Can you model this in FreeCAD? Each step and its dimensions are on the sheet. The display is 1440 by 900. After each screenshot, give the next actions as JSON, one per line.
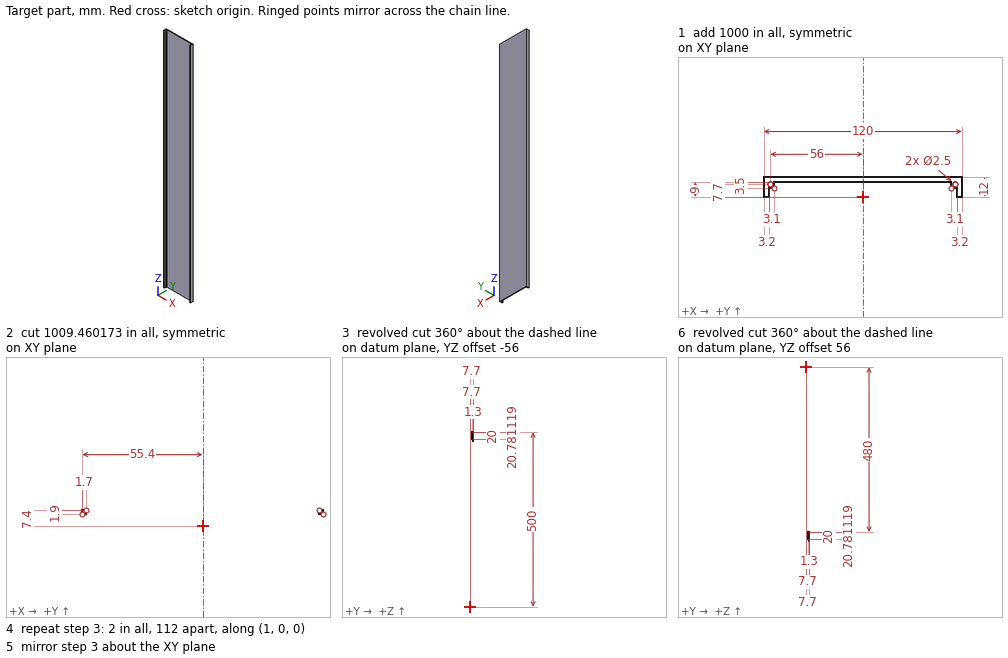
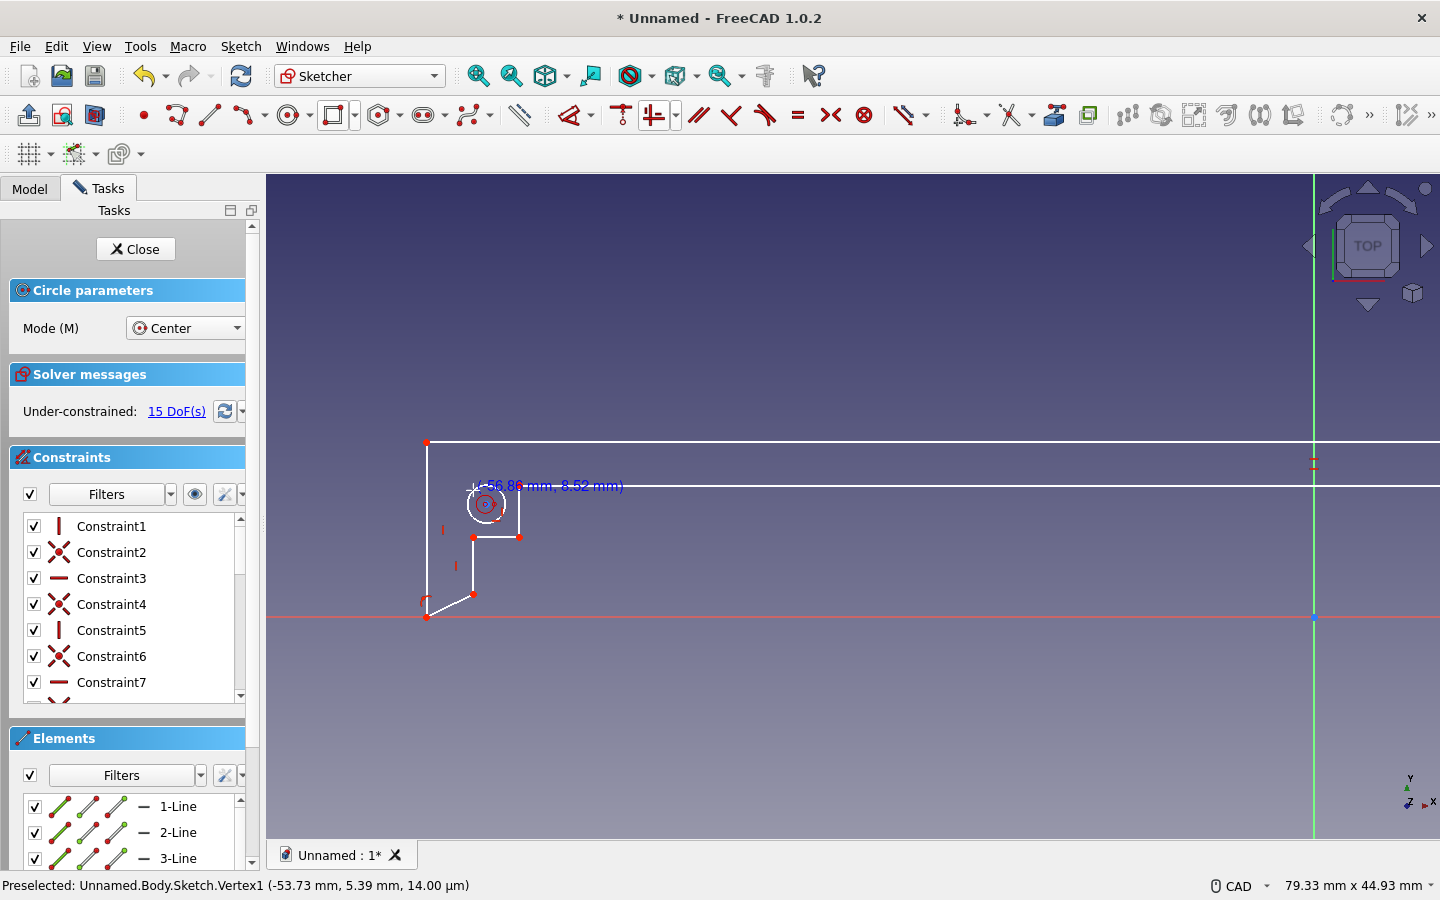
{"action": "scroll", "coordinate": [476, 494], "scroll_direction": "down", "scroll_amount": 5}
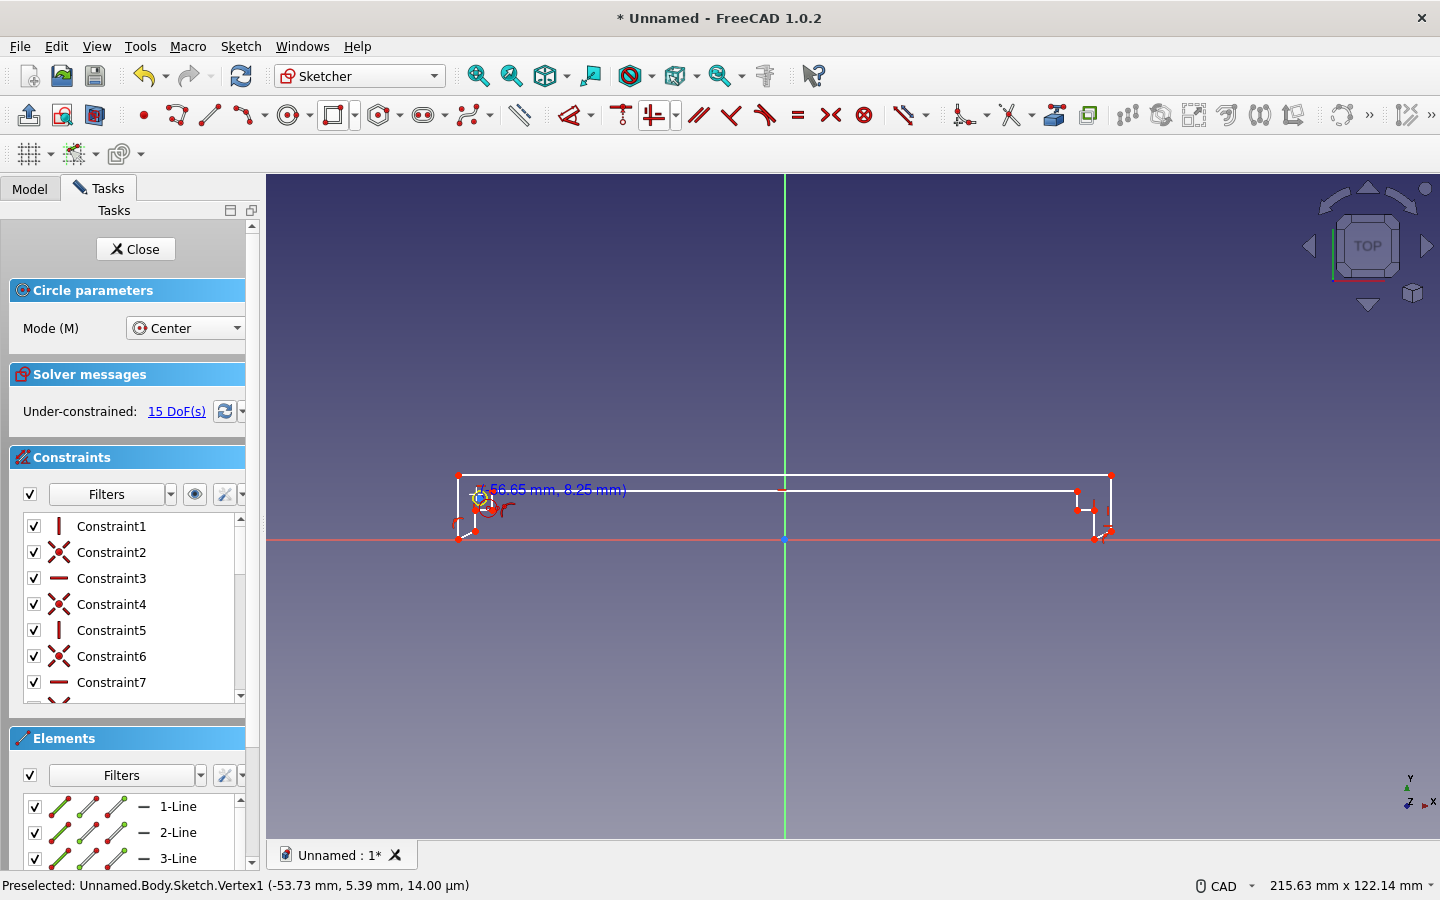
{"action": "scroll", "coordinate": [1089, 498], "scroll_direction": "up", "scroll_amount": 7}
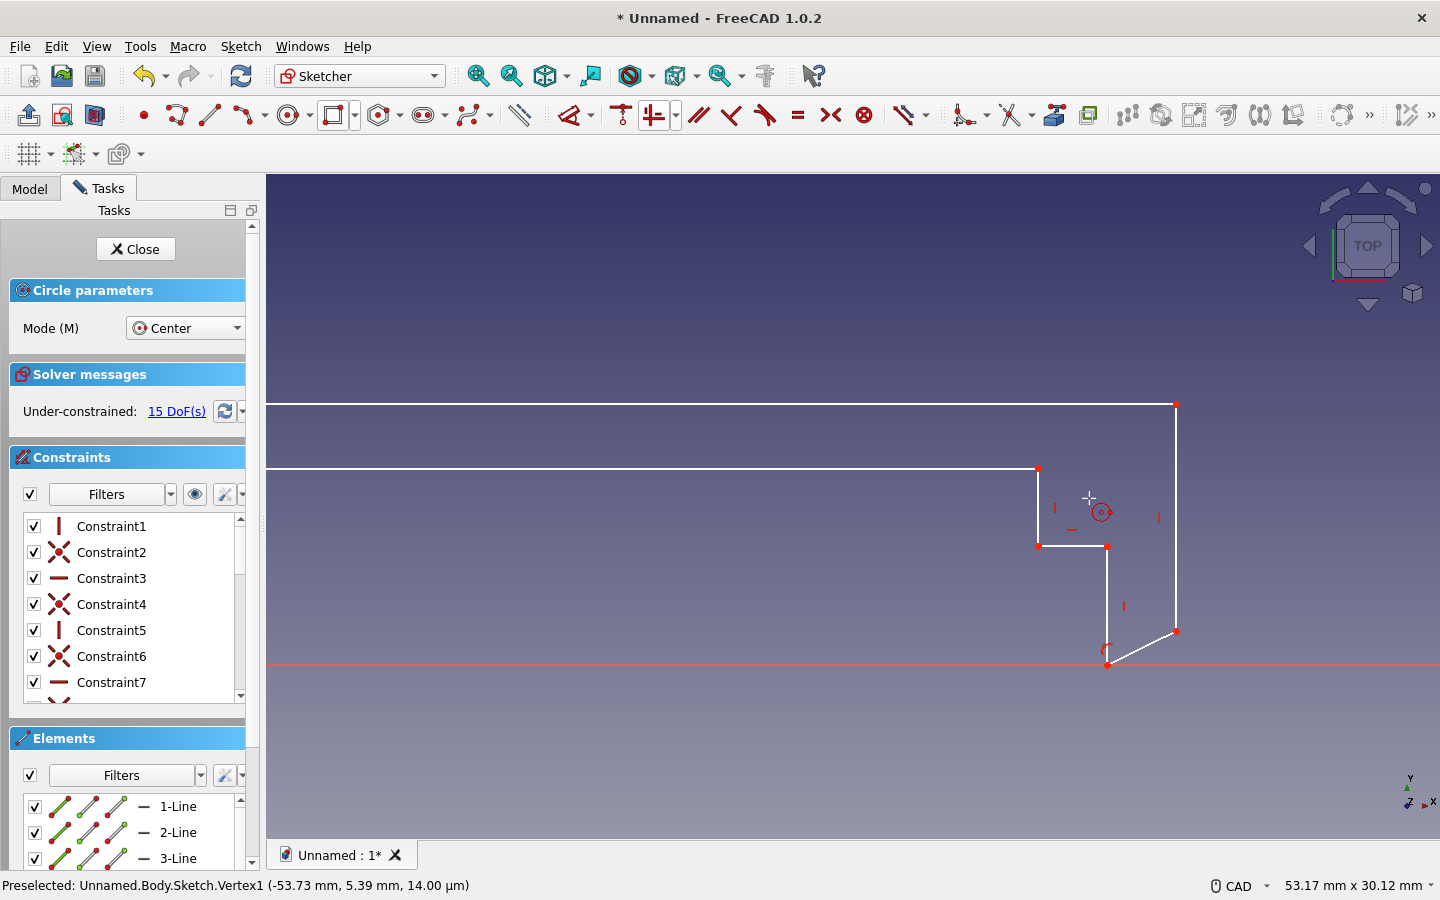
{"action": "scroll", "coordinate": [1090, 498], "scroll_direction": "down", "scroll_amount": 7}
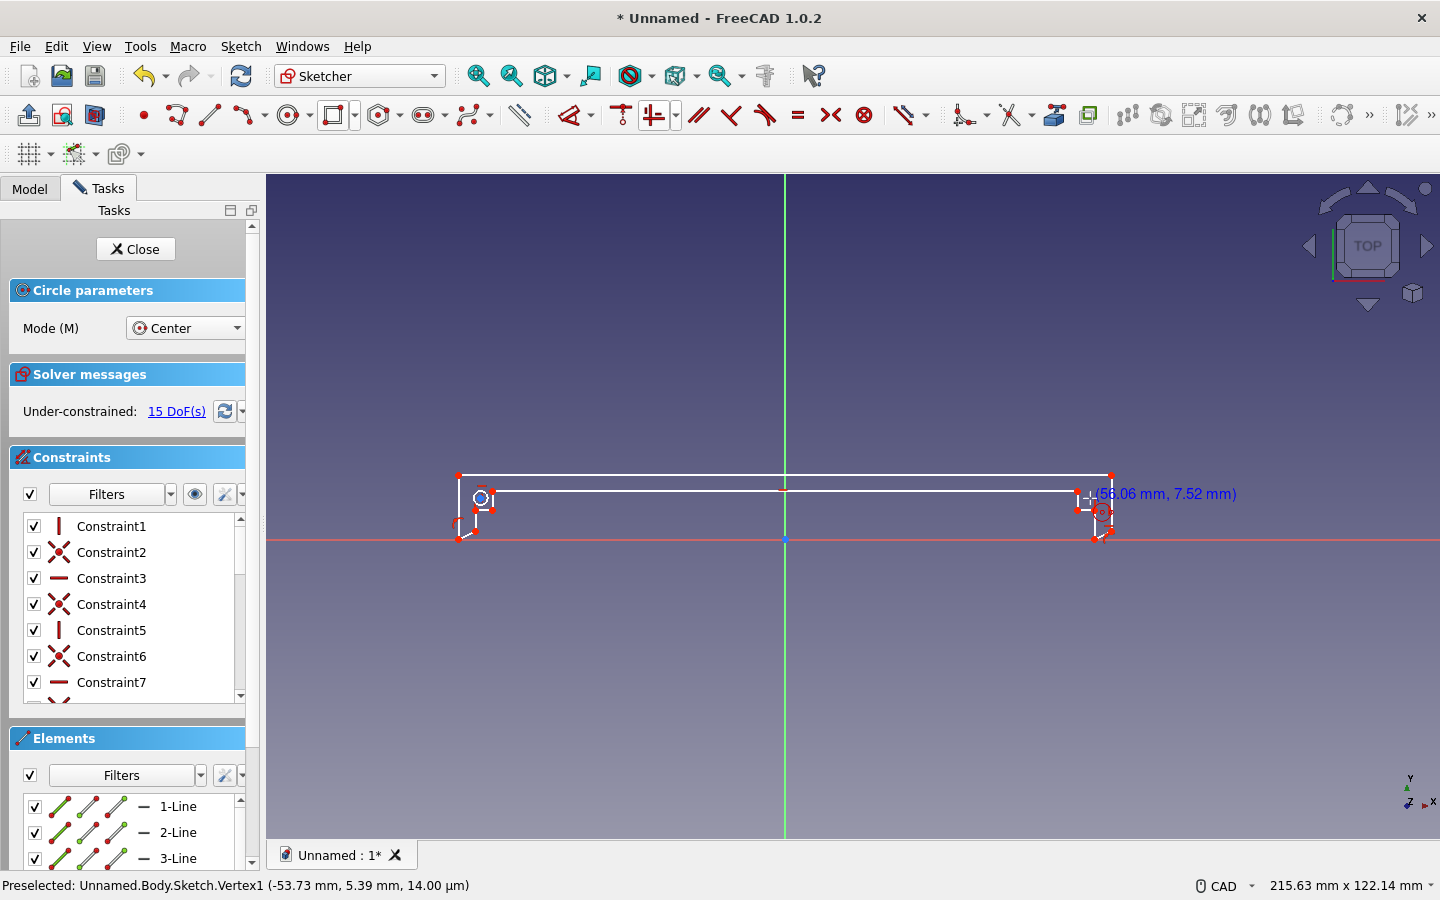
{"action": "scroll", "coordinate": [1090, 498], "scroll_direction": "up", "scroll_amount": 2}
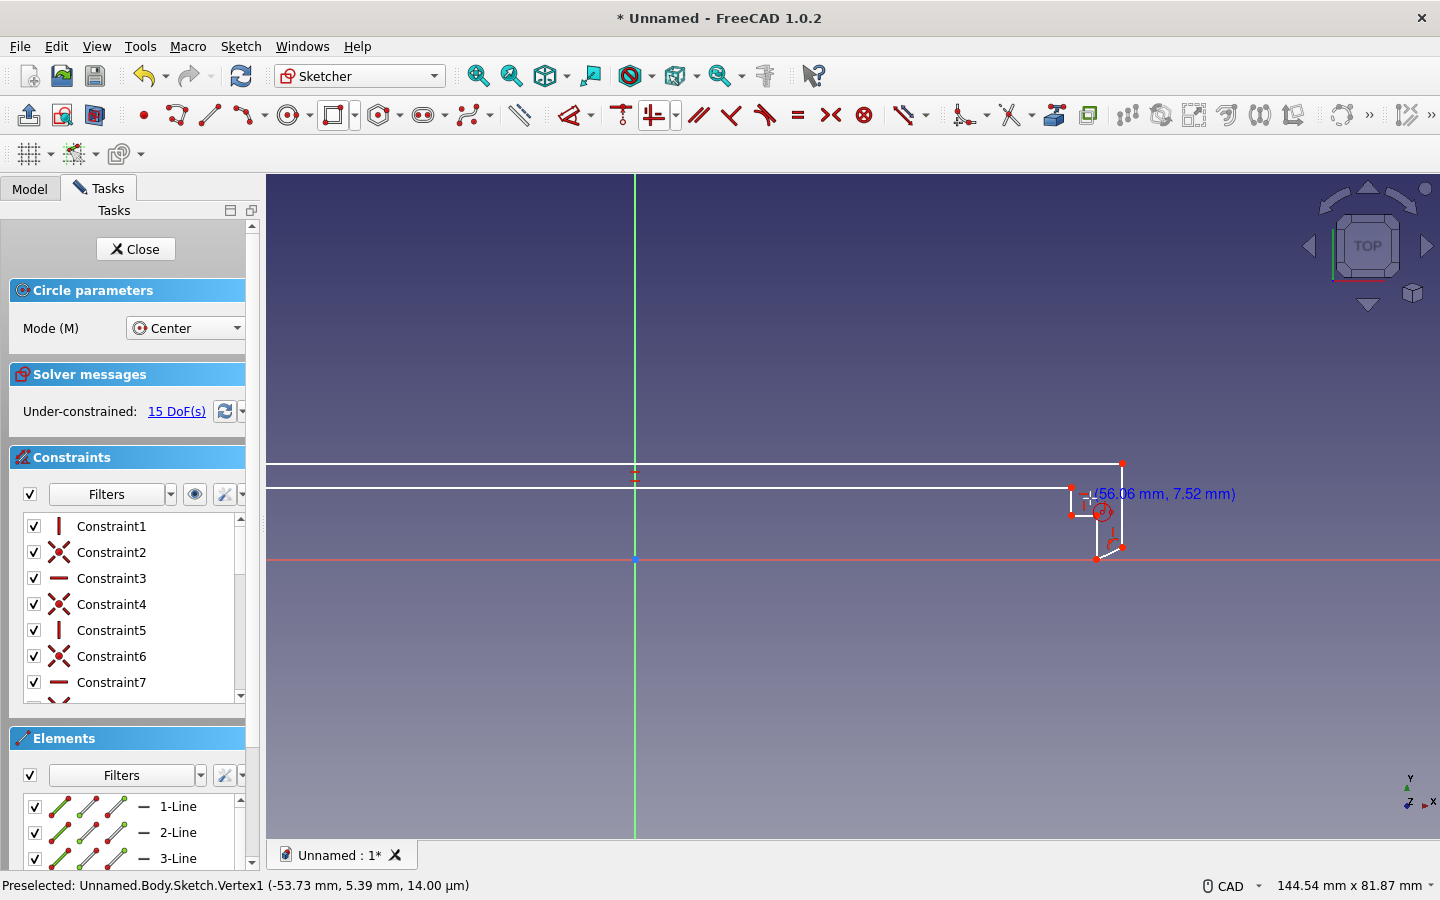
{"action": "left_click", "coordinate": [1090, 497]}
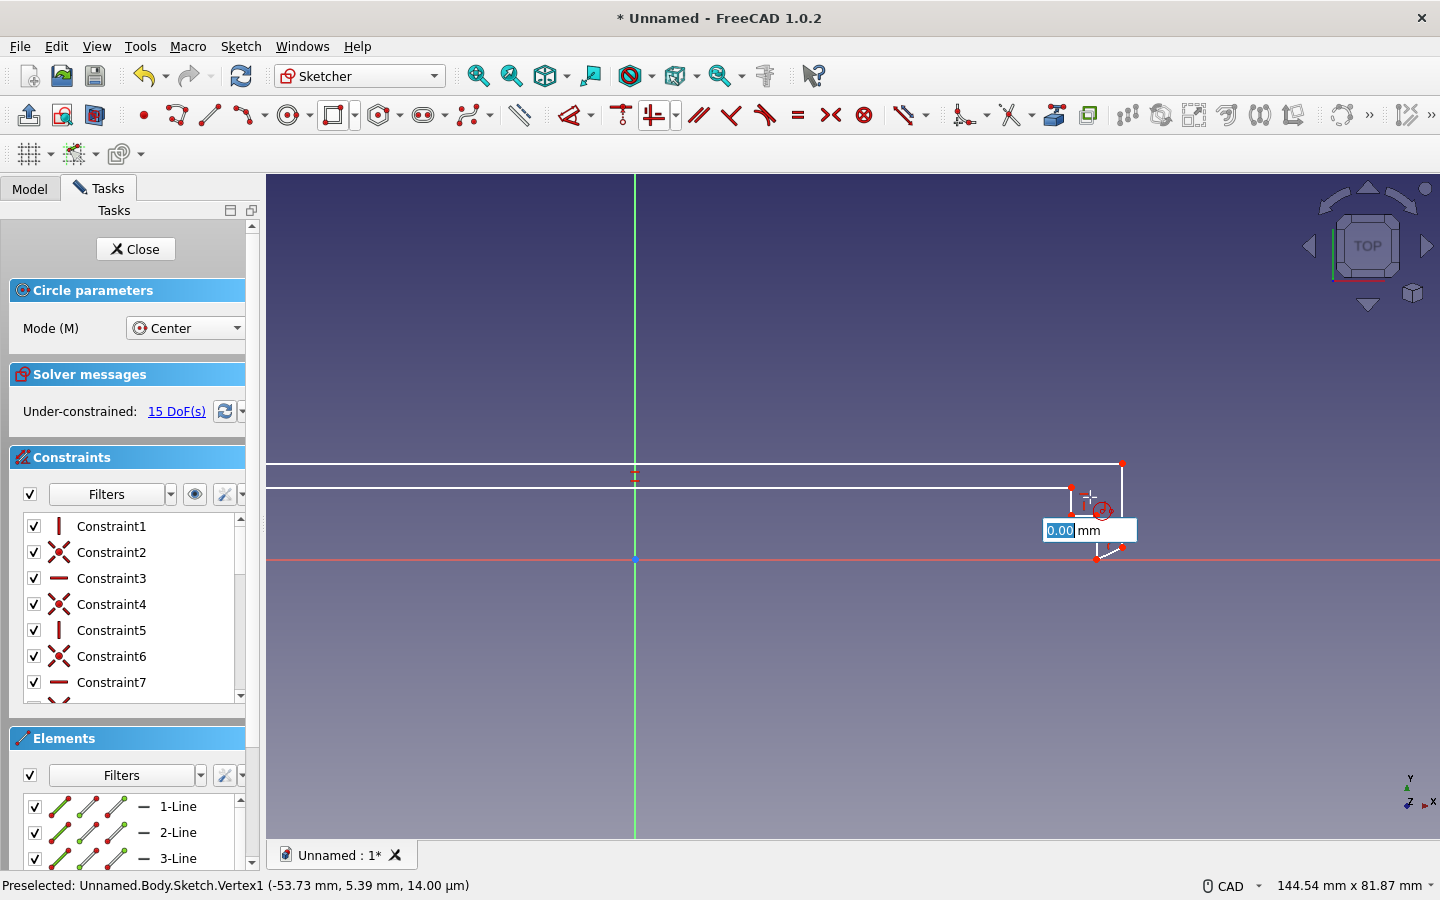
{"action": "scroll", "coordinate": [1097, 490], "scroll_direction": "up", "scroll_amount": 3}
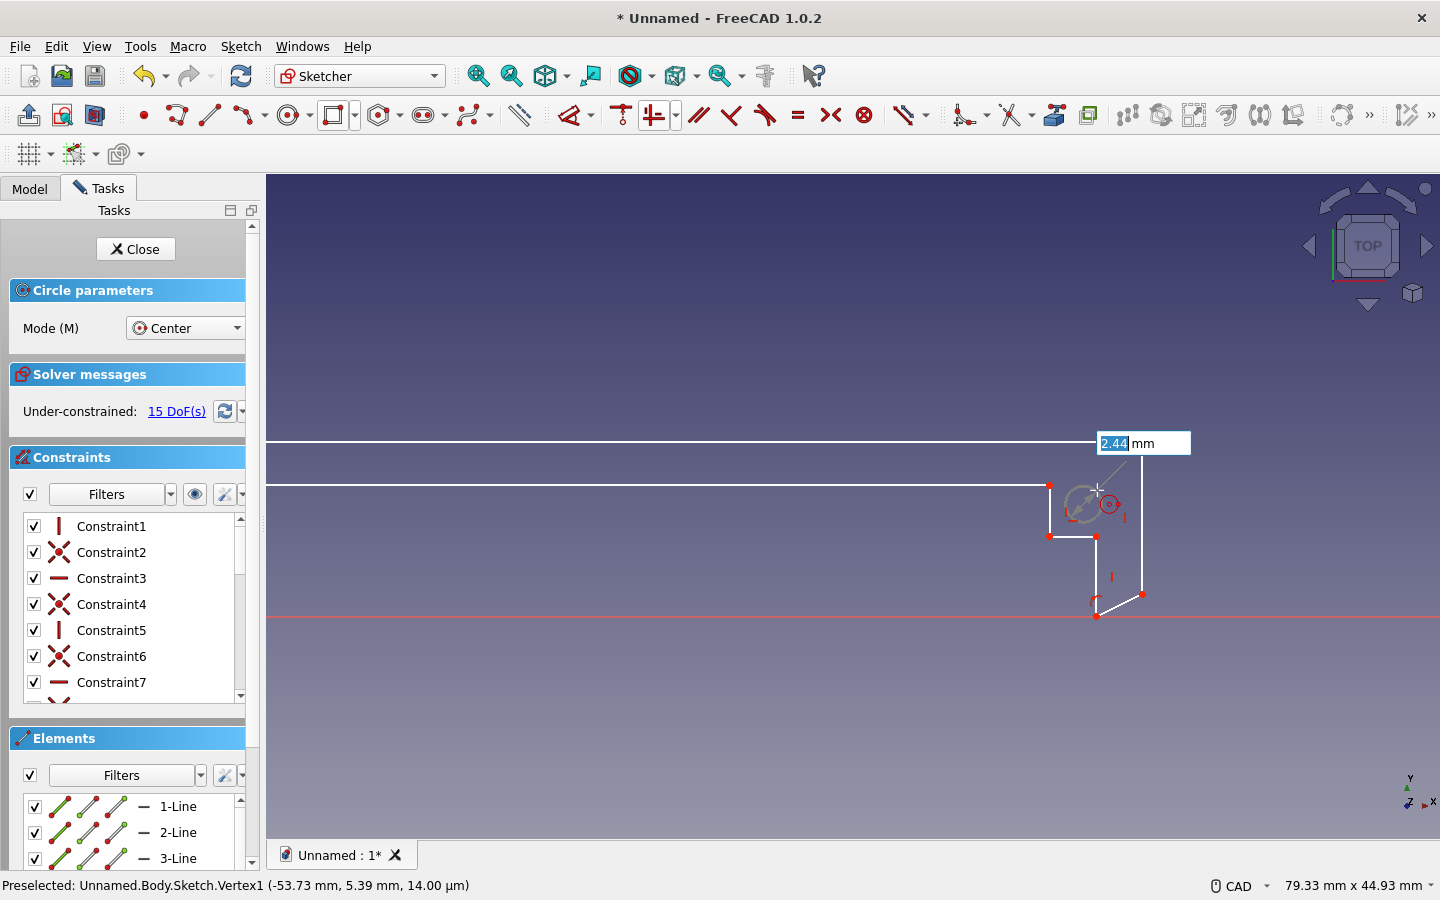
{"action": "left_click", "coordinate": [1097, 490]}
{"action": "key", "text": "Escape"}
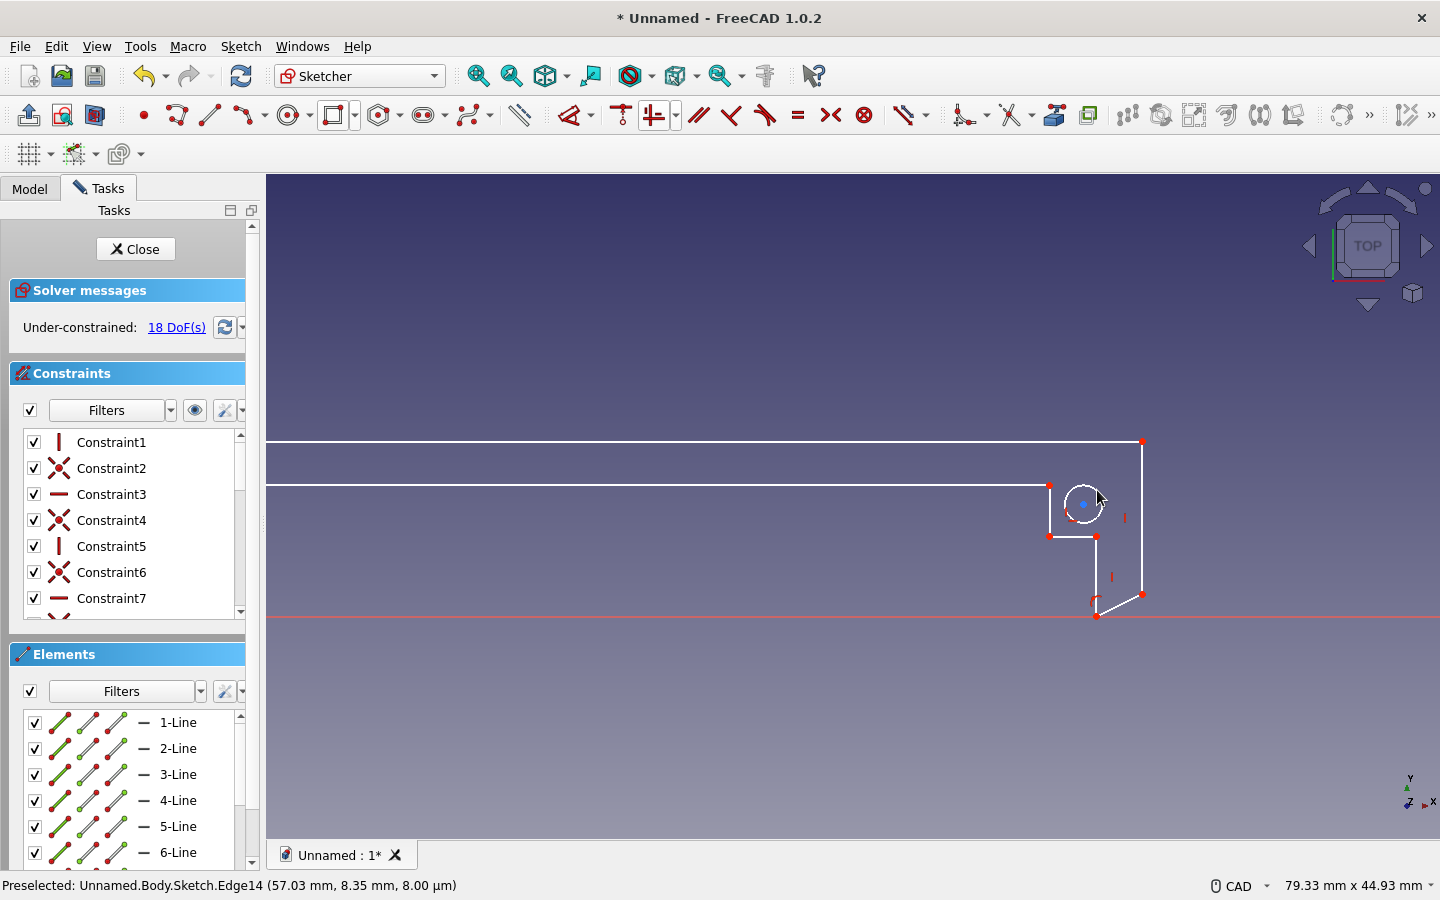
{"action": "left_click", "coordinate": [1128, 601]}